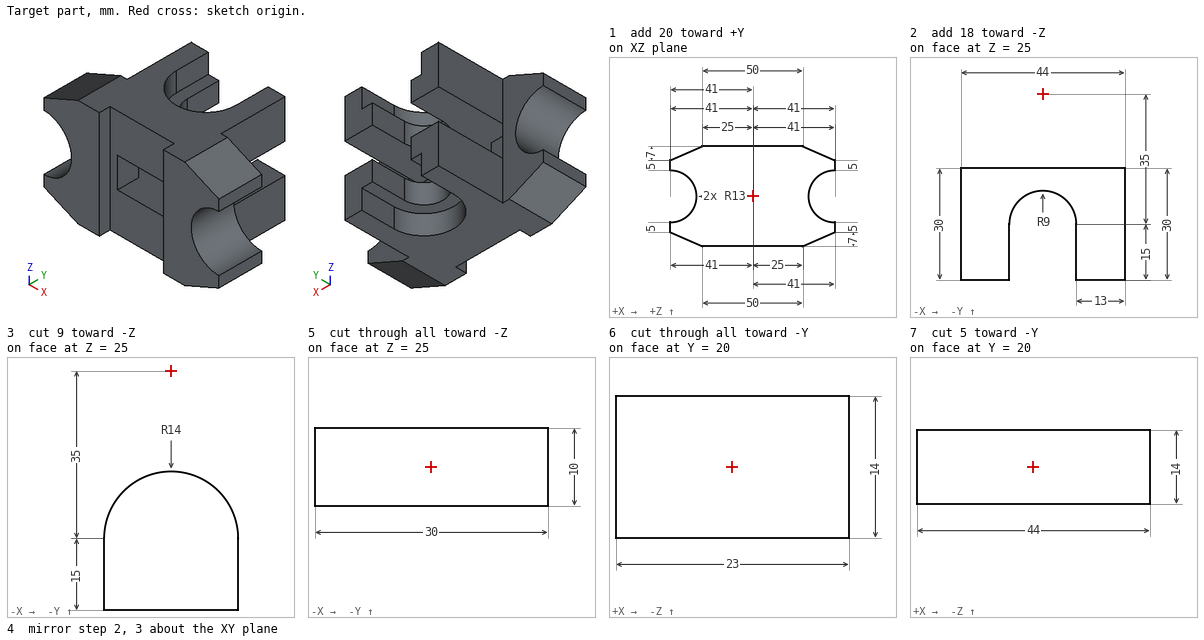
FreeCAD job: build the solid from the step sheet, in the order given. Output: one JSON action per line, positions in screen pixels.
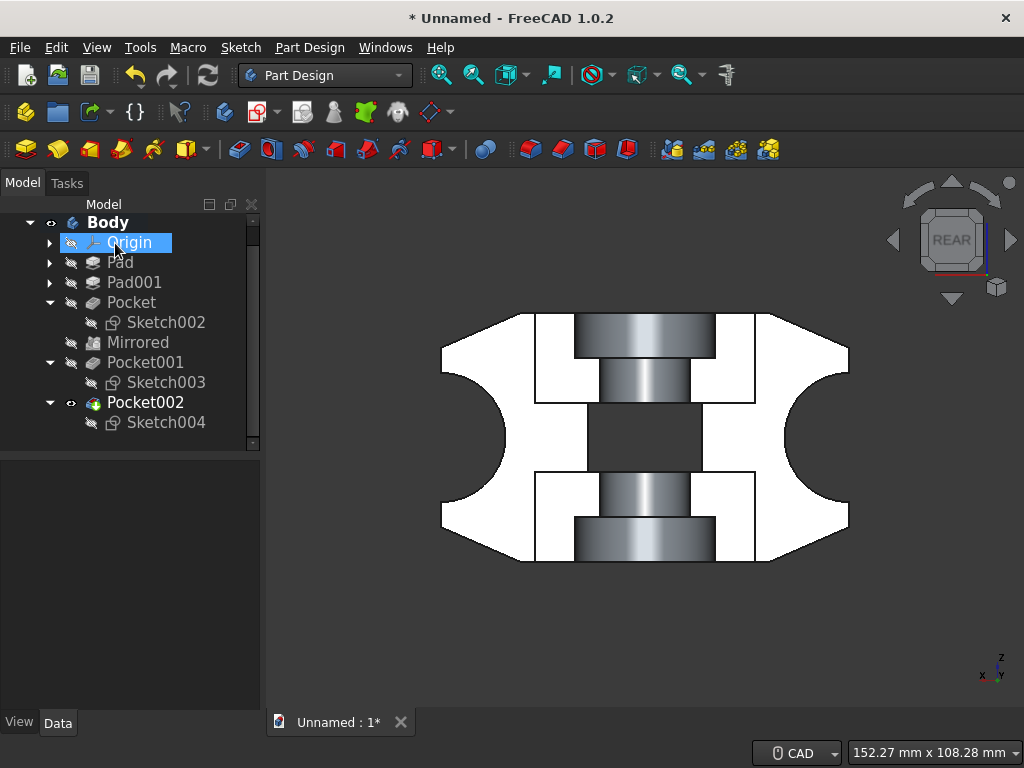
{"action": "left_click", "coordinate": [734, 437]}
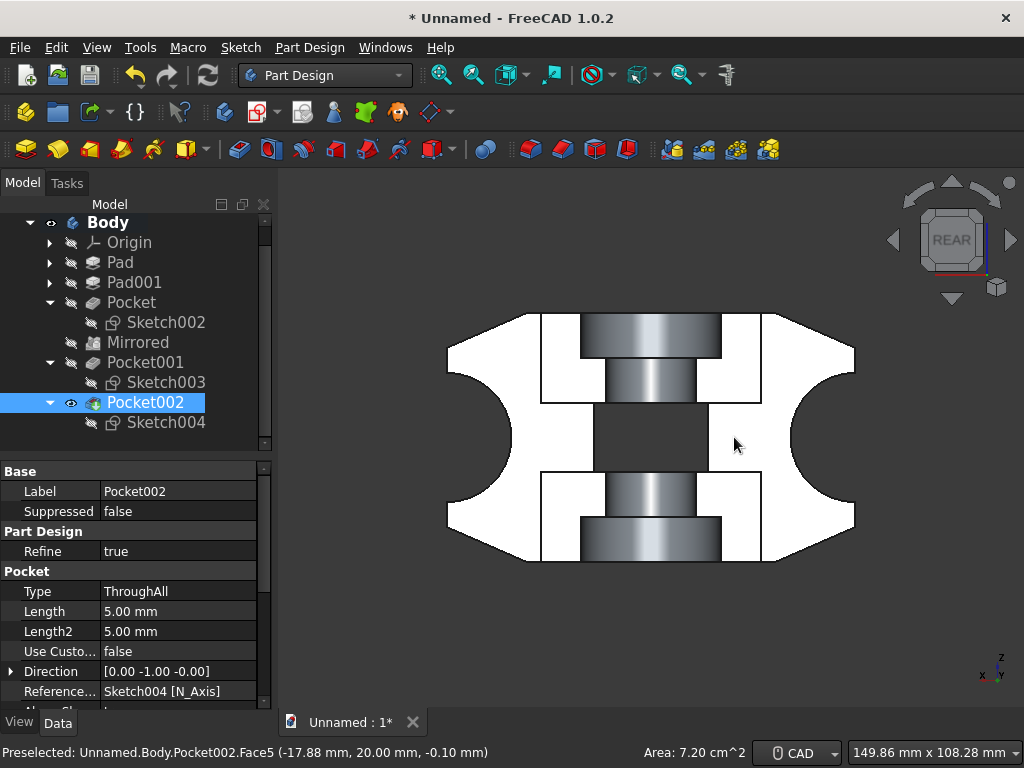
{"action": "left_click", "coordinate": [258, 112]}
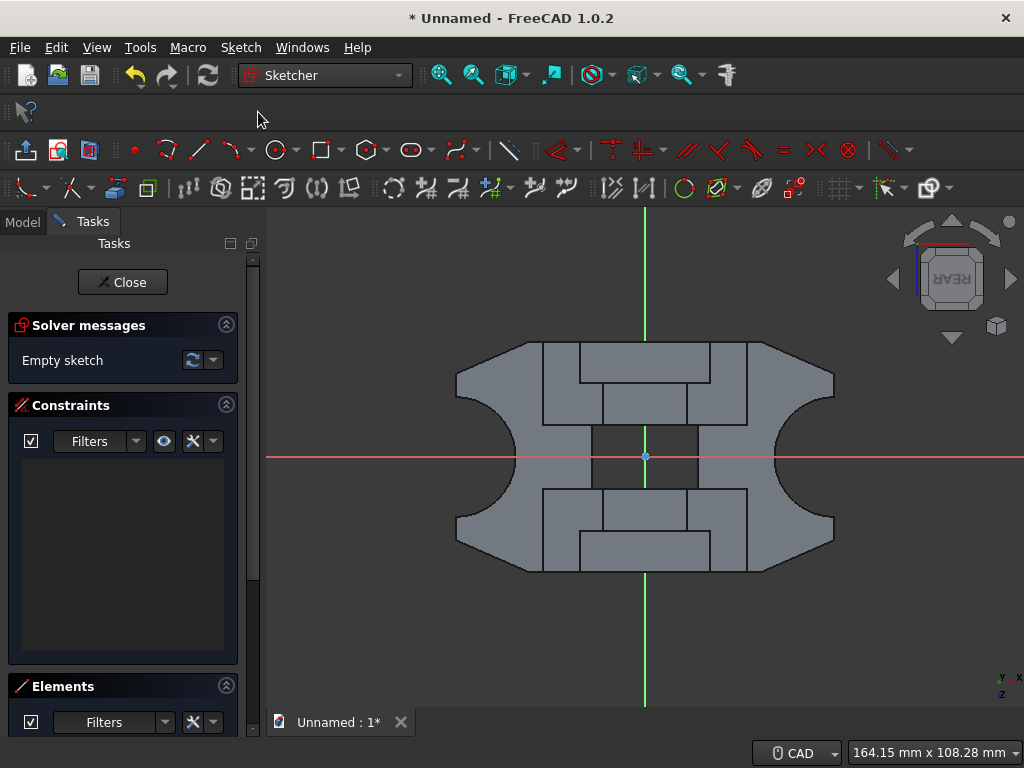
{"action": "scroll", "coordinate": [728, 457], "scroll_direction": "up", "scroll_amount": 3}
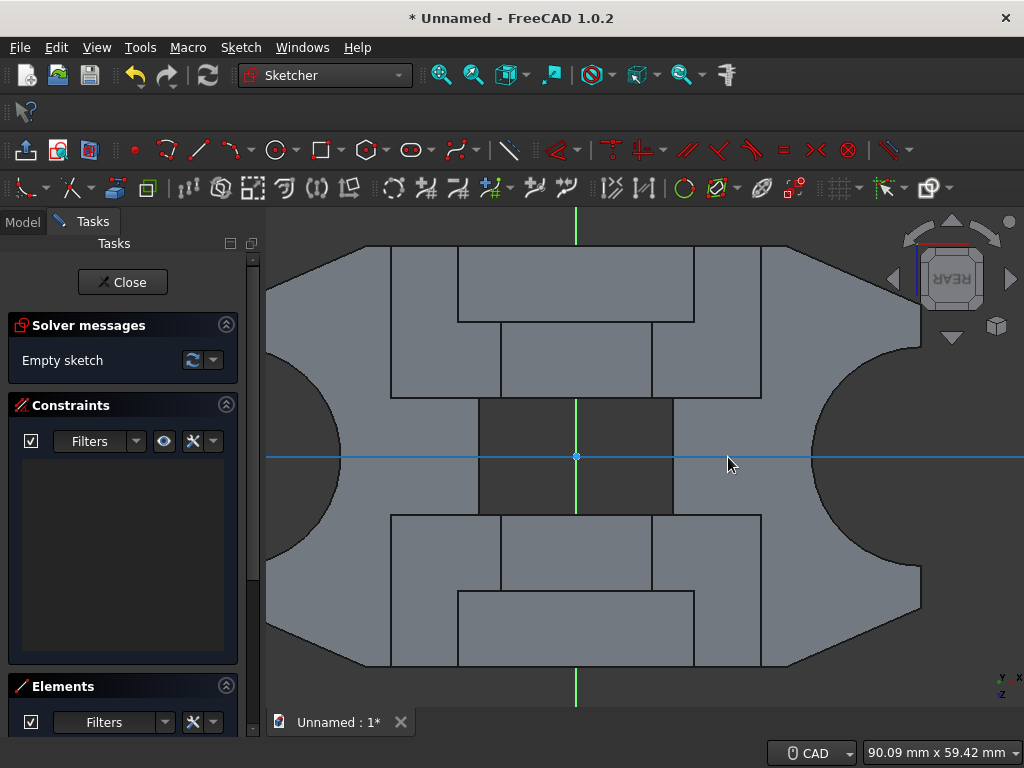
{"action": "left_click", "coordinate": [344, 150]}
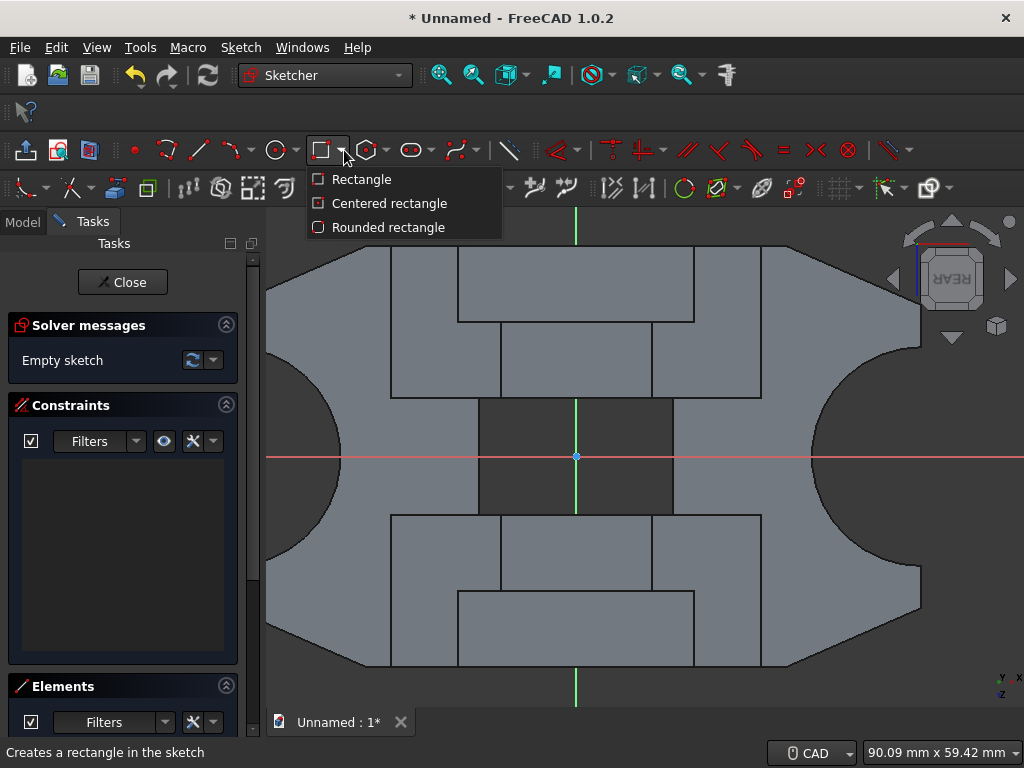
{"action": "left_click", "coordinate": [404, 203]}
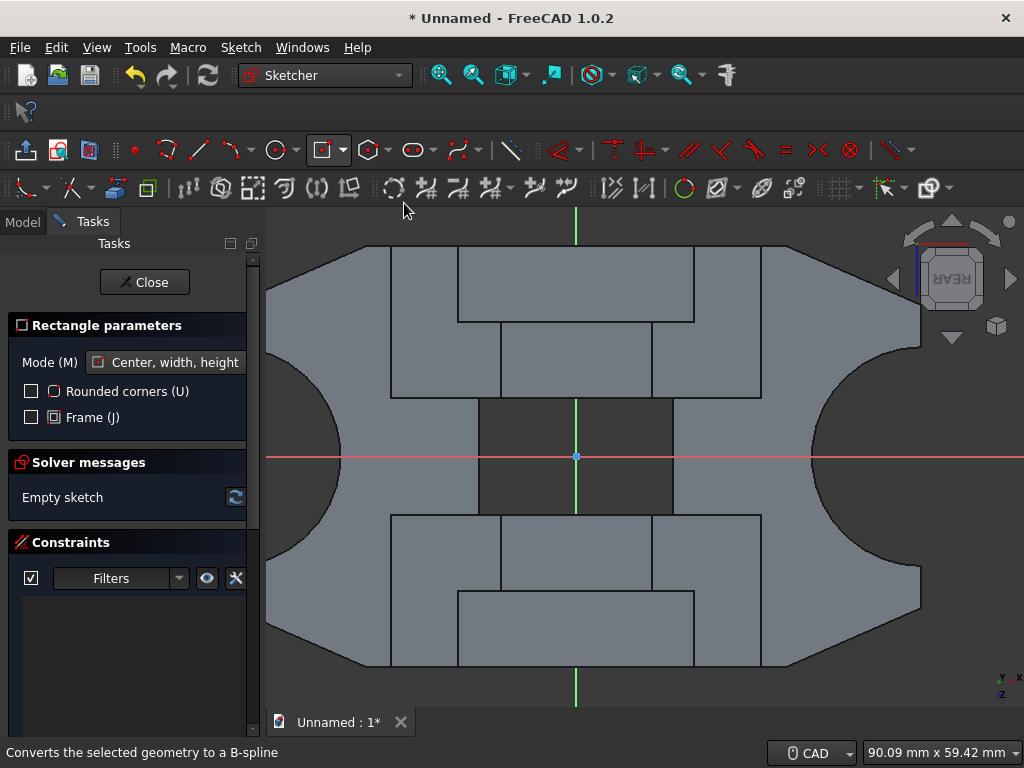
{"action": "left_click", "coordinate": [576, 457]}
{"action": "mouse_move", "coordinate": [761, 398]}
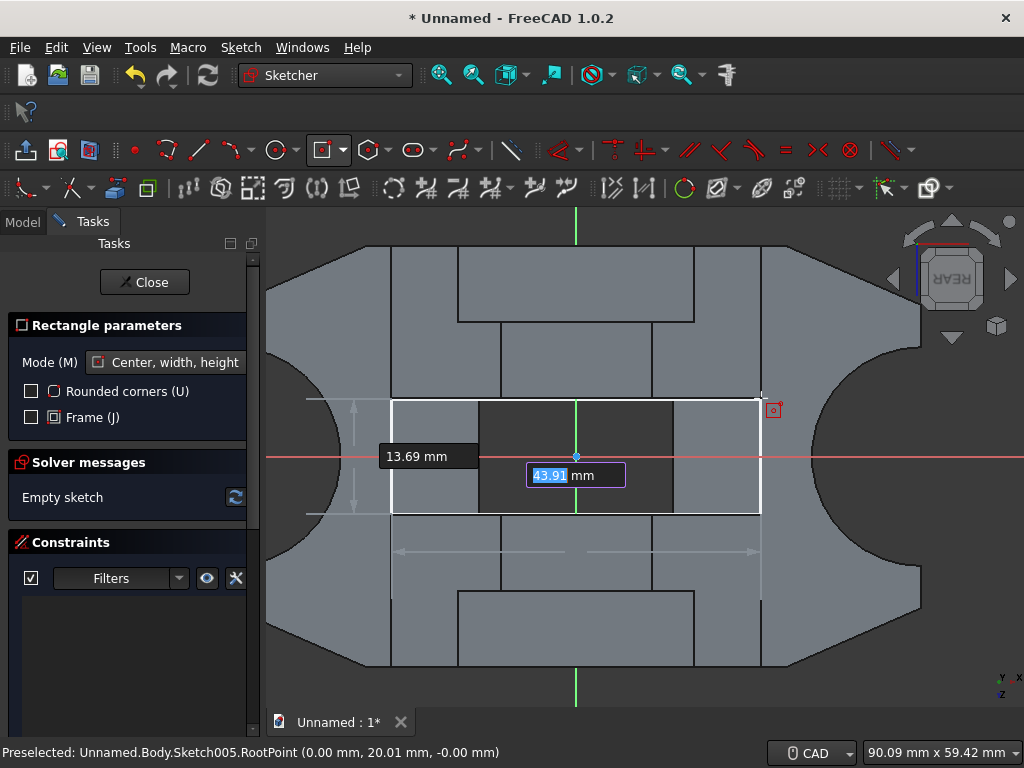
{"action": "type", "text": "44"}
{"action": "key", "text": "Tab"}
{"action": "type", "text": "14"}
{"action": "key", "text": "Return"}
{"action": "key", "text": "Escape"}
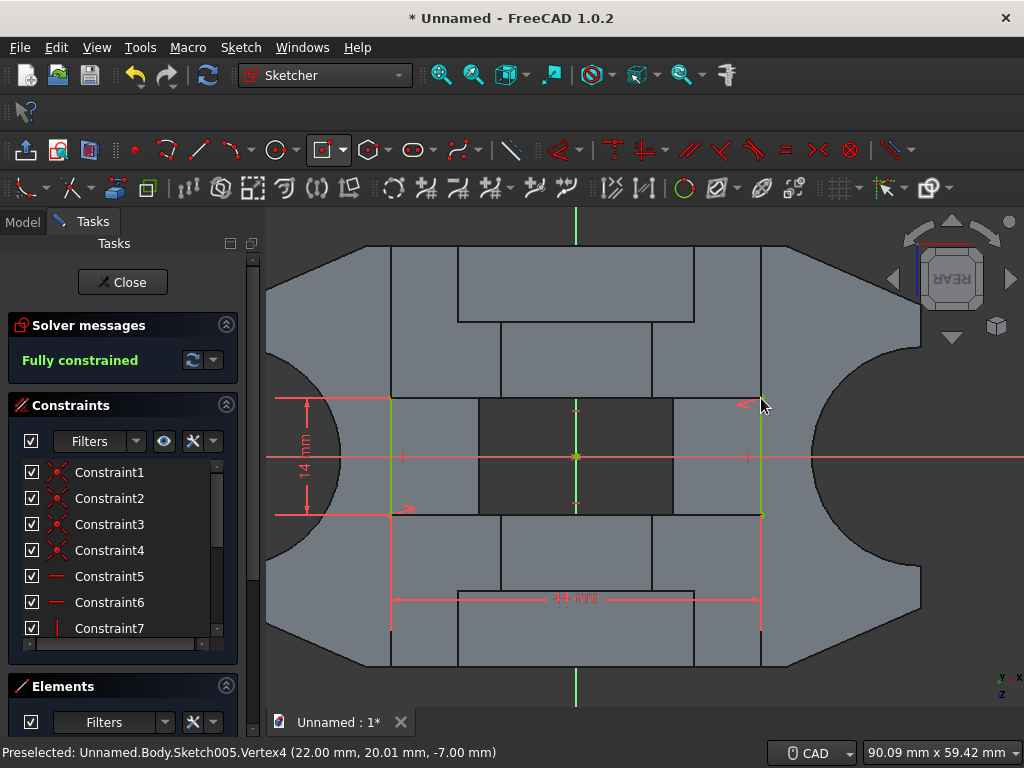
{"action": "left_click", "coordinate": [123, 282]}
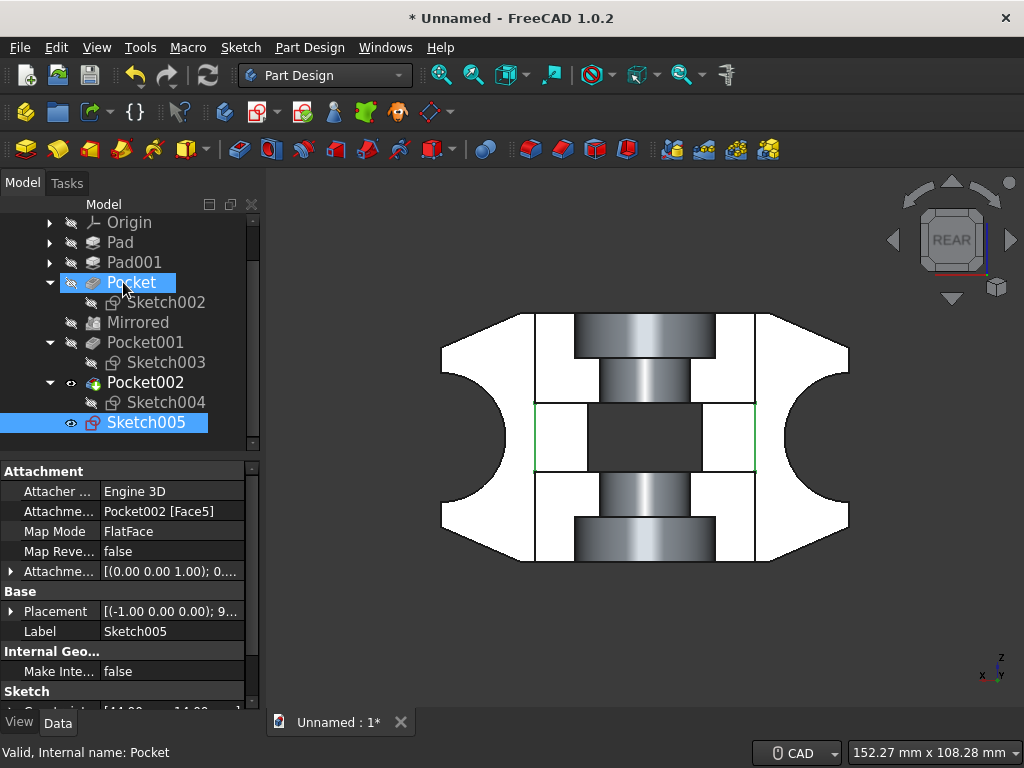
{"action": "left_click", "coordinate": [240, 150]}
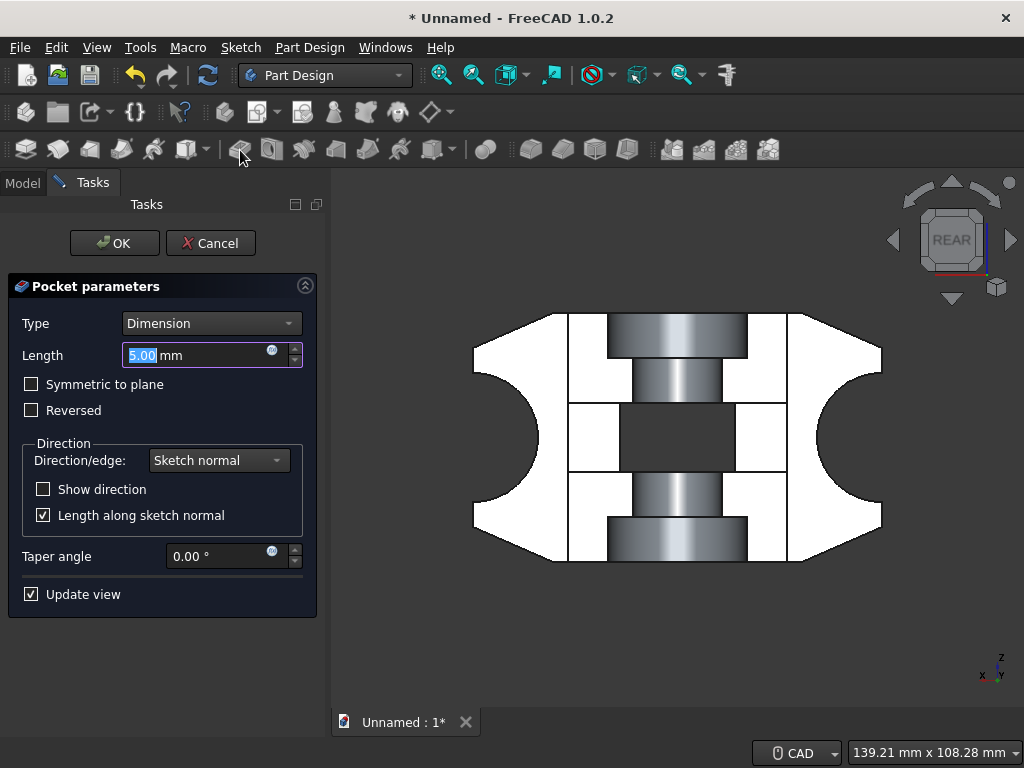
{"action": "type", "text": "5"}
{"action": "key", "text": "Tab"}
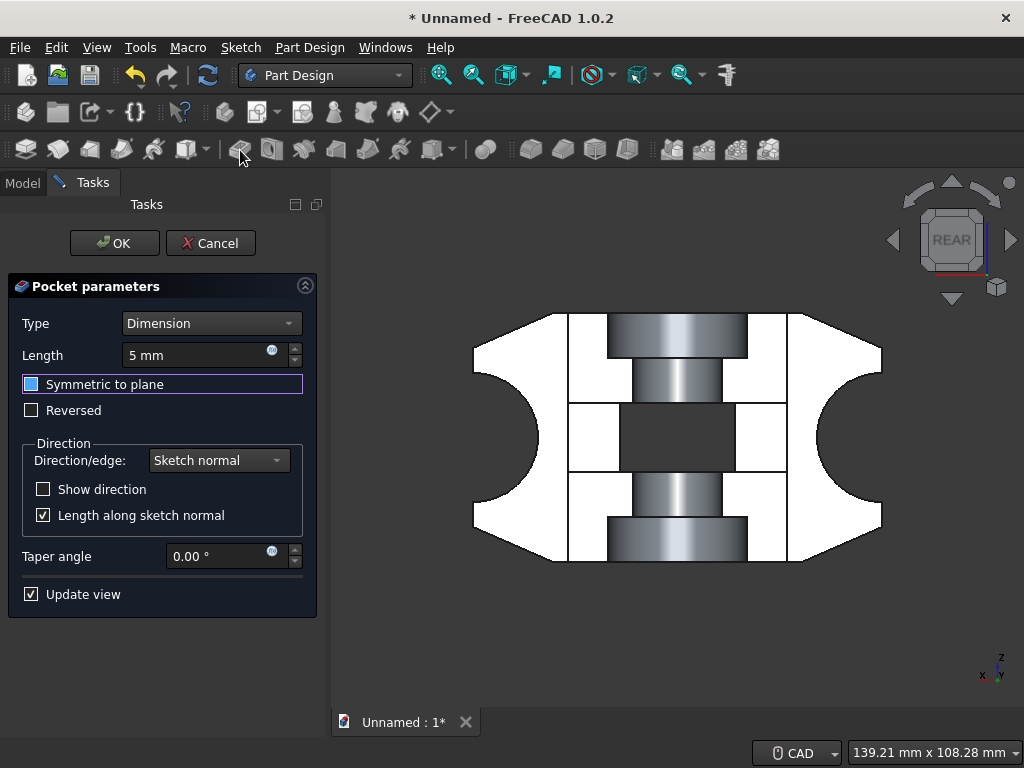
{"action": "left_click", "coordinate": [115, 243]}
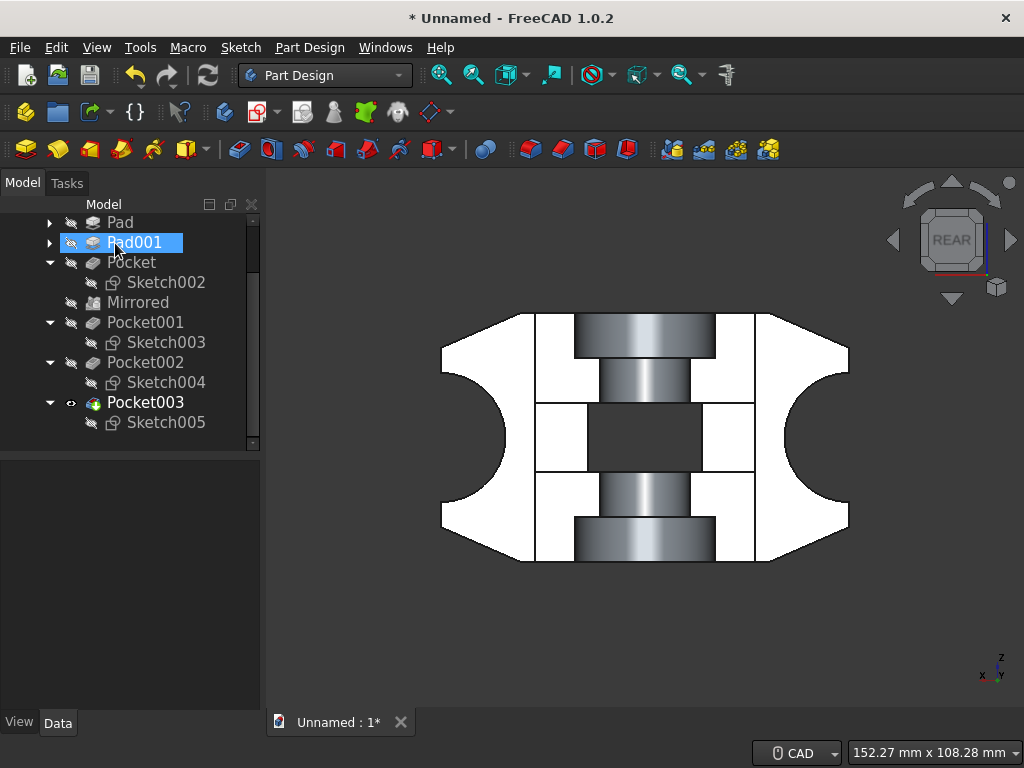
{"action": "key", "text": "0"}